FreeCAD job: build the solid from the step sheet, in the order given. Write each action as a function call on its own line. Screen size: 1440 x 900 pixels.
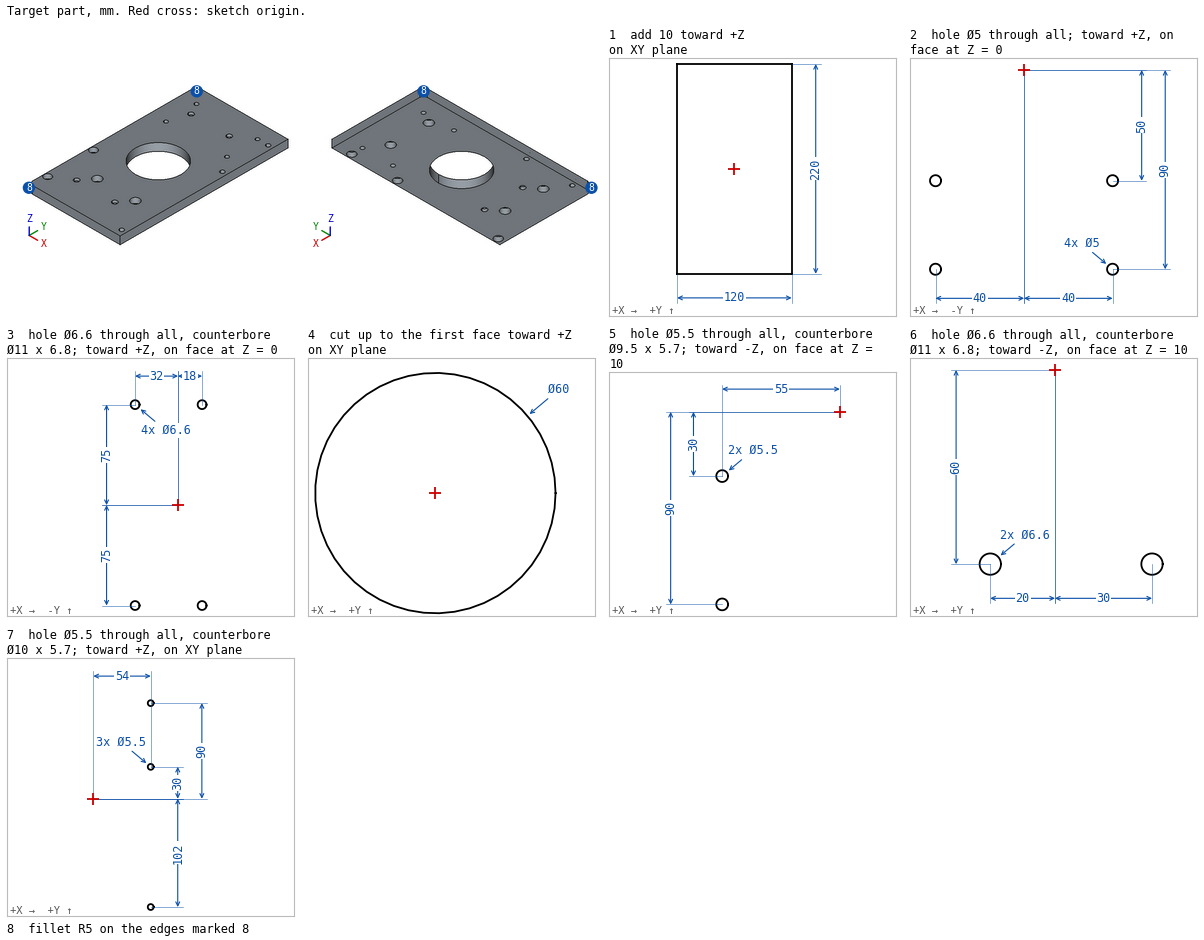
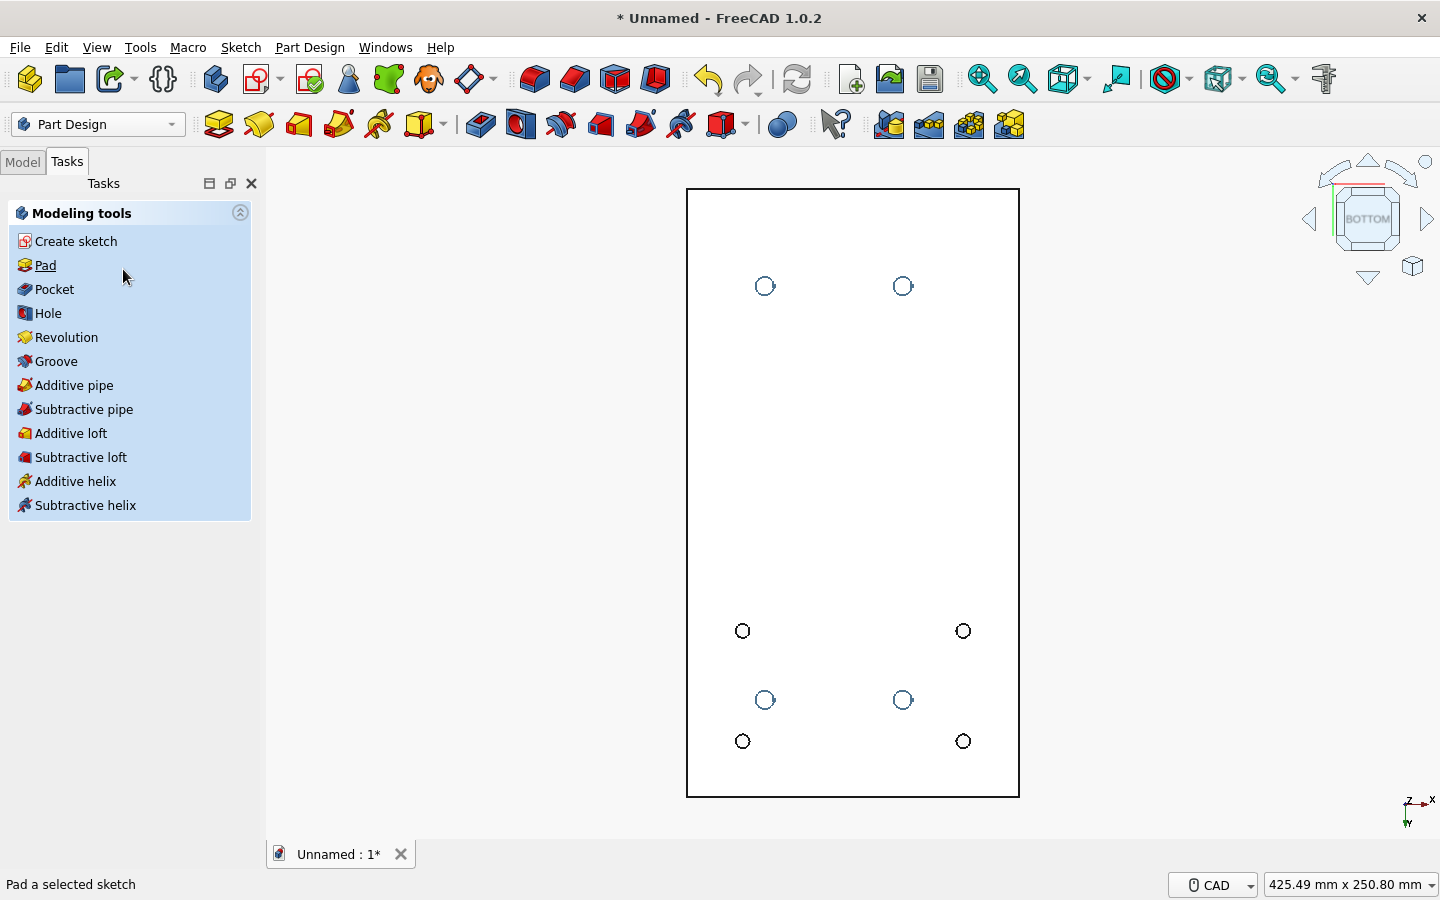
click(522, 124)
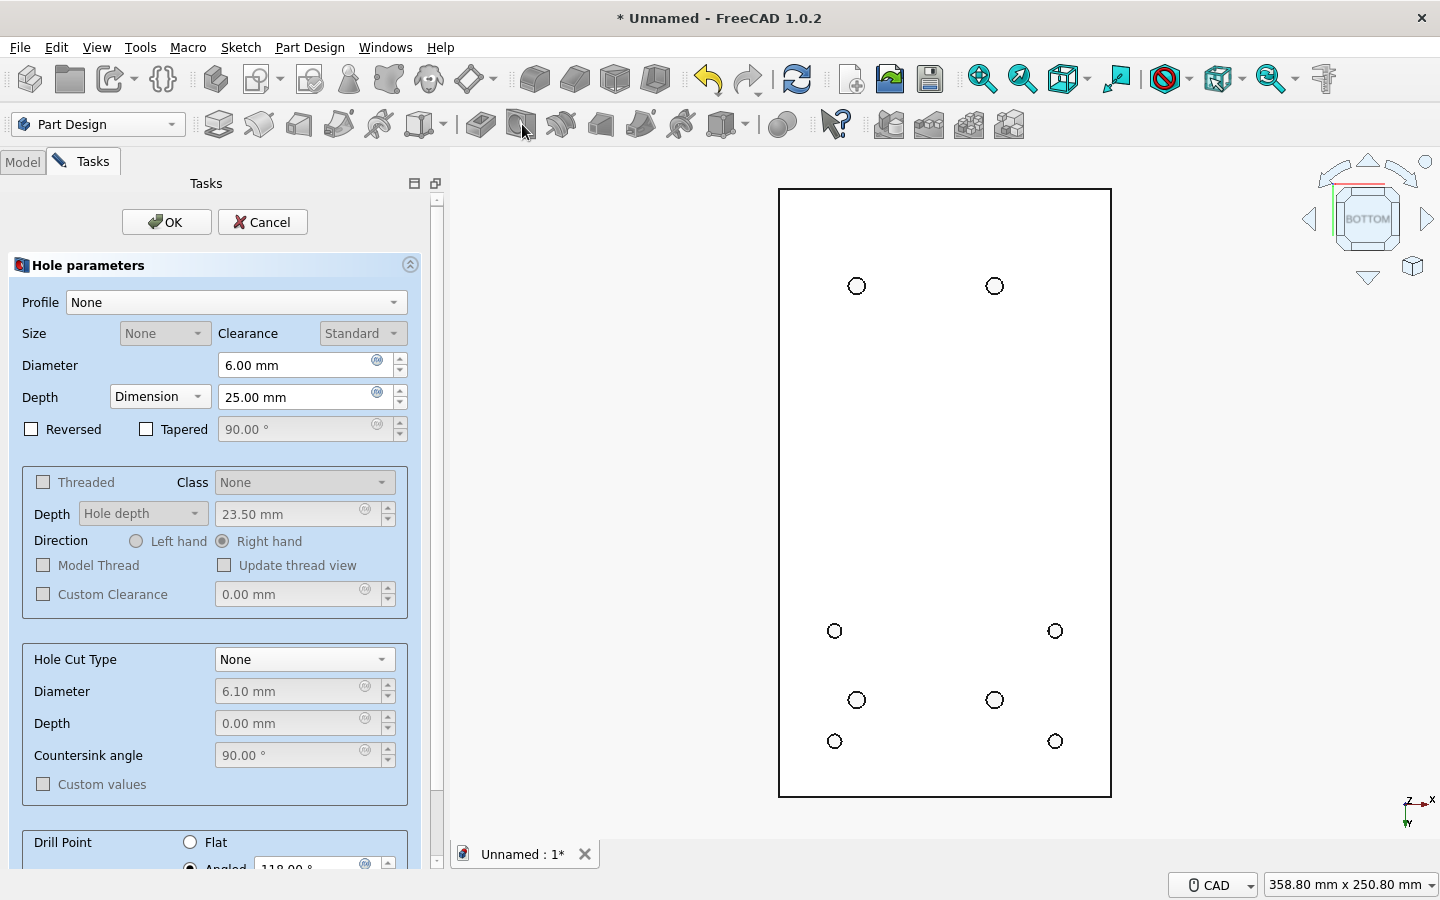
triple_click(305, 365)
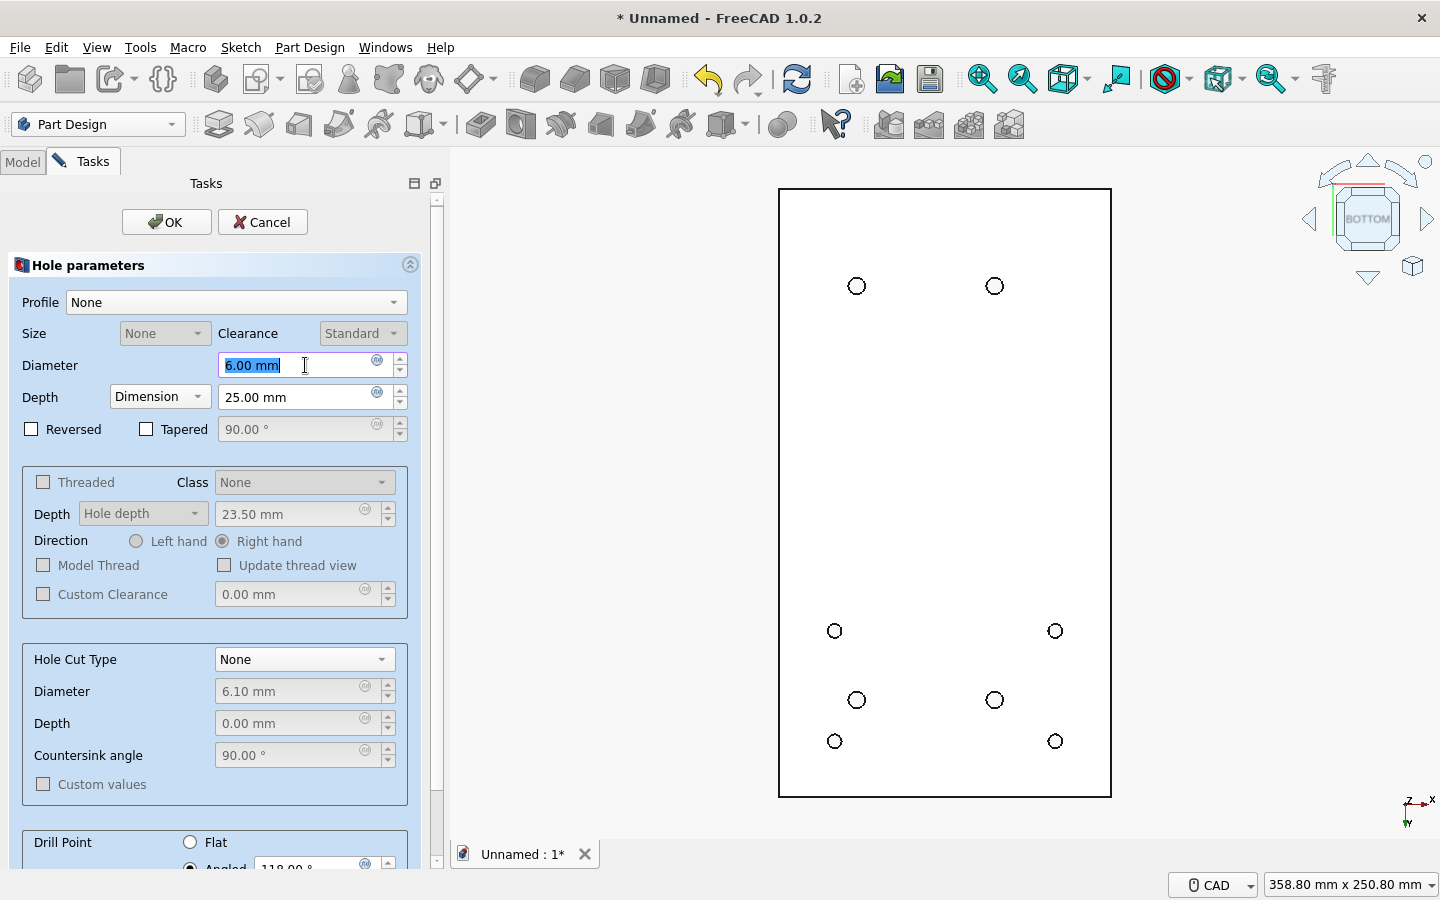
text(6.6)
key(Tab)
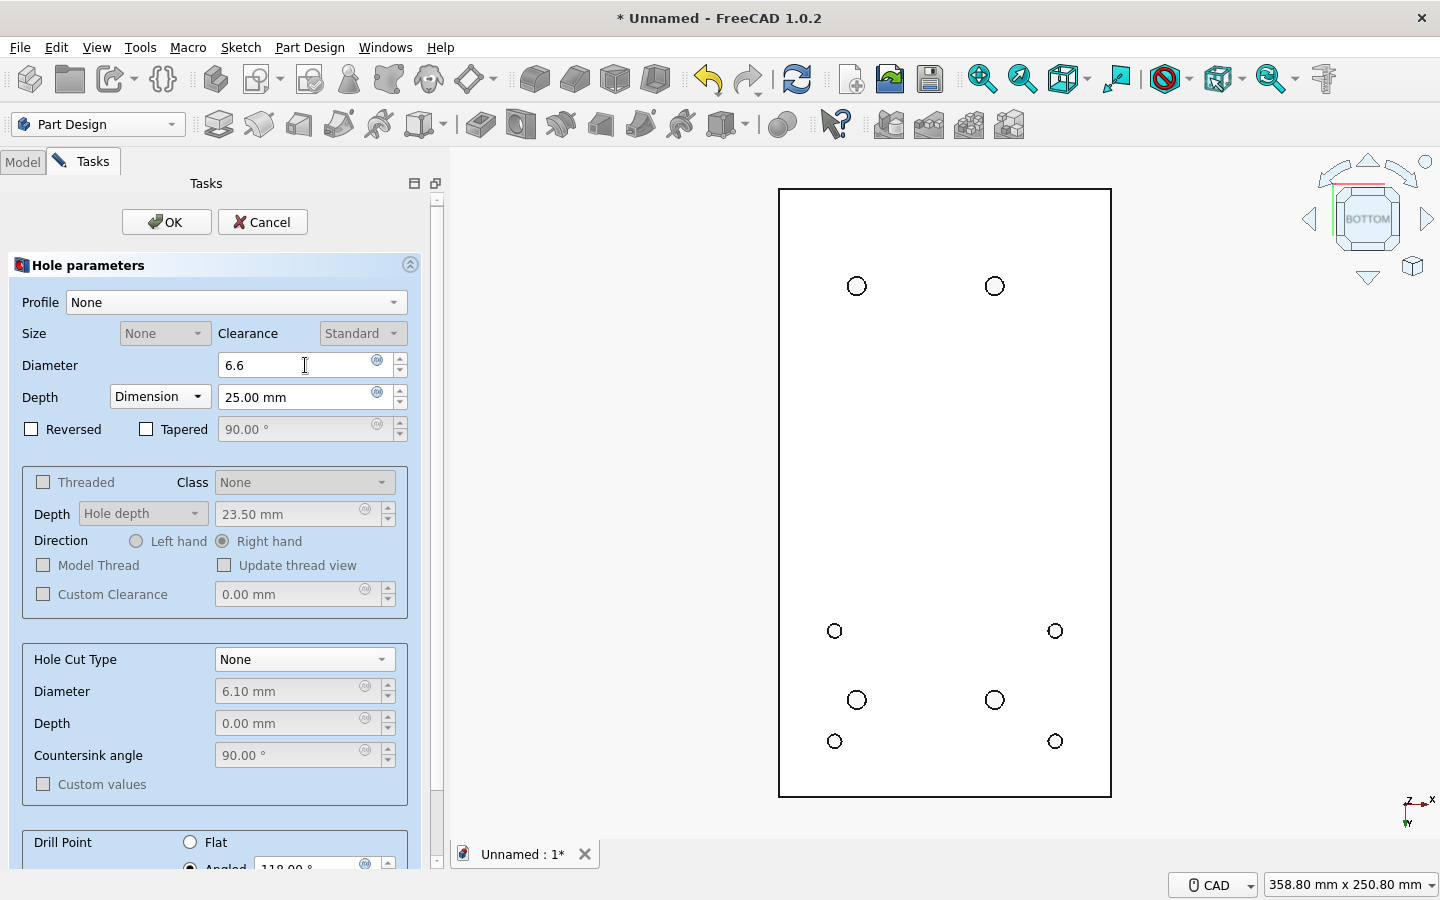
click(161, 396)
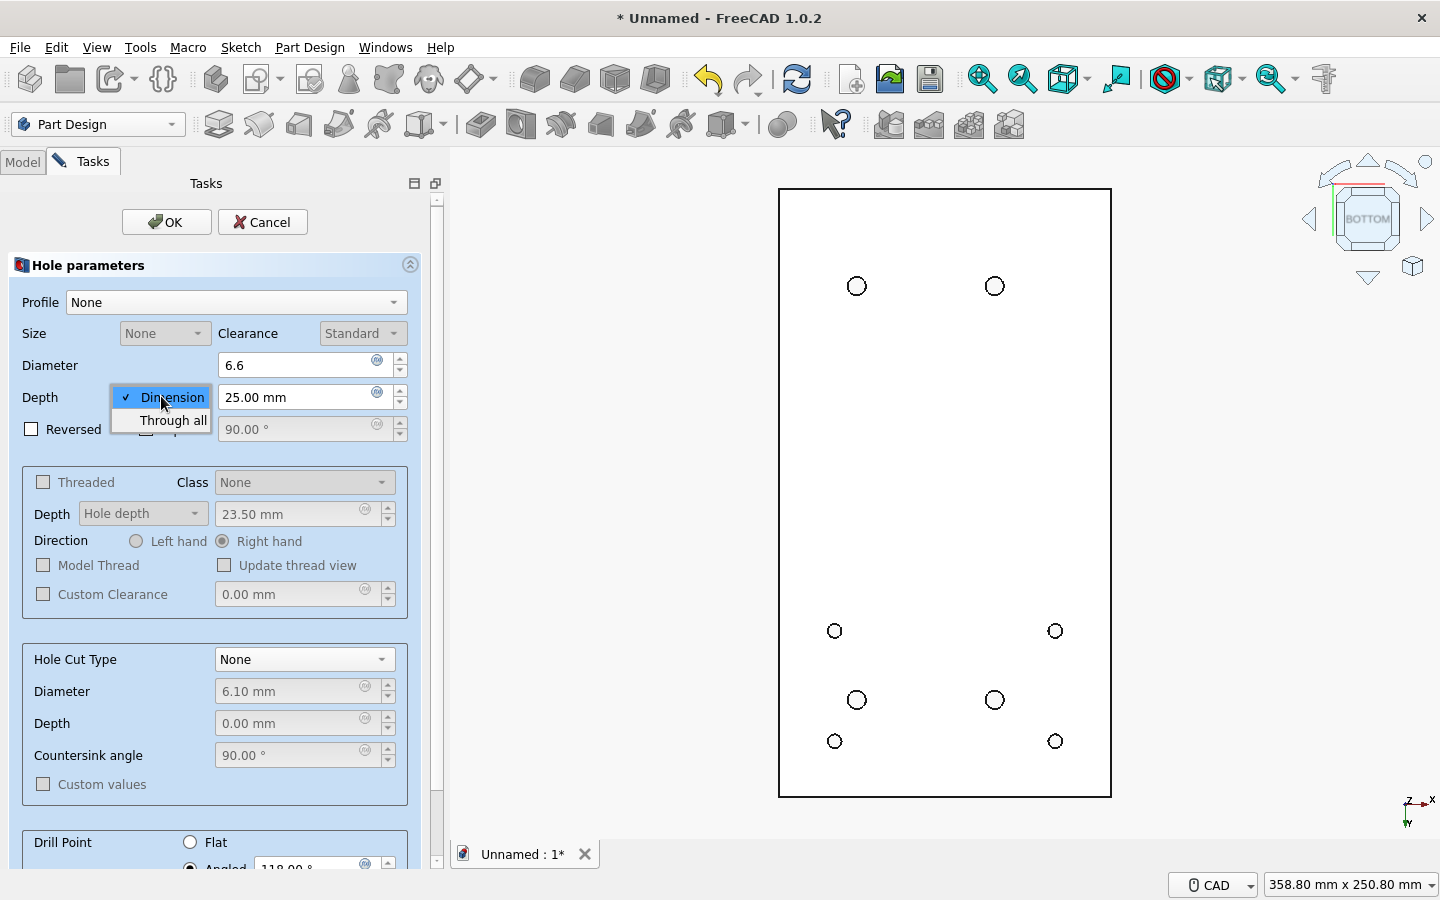
click(160, 420)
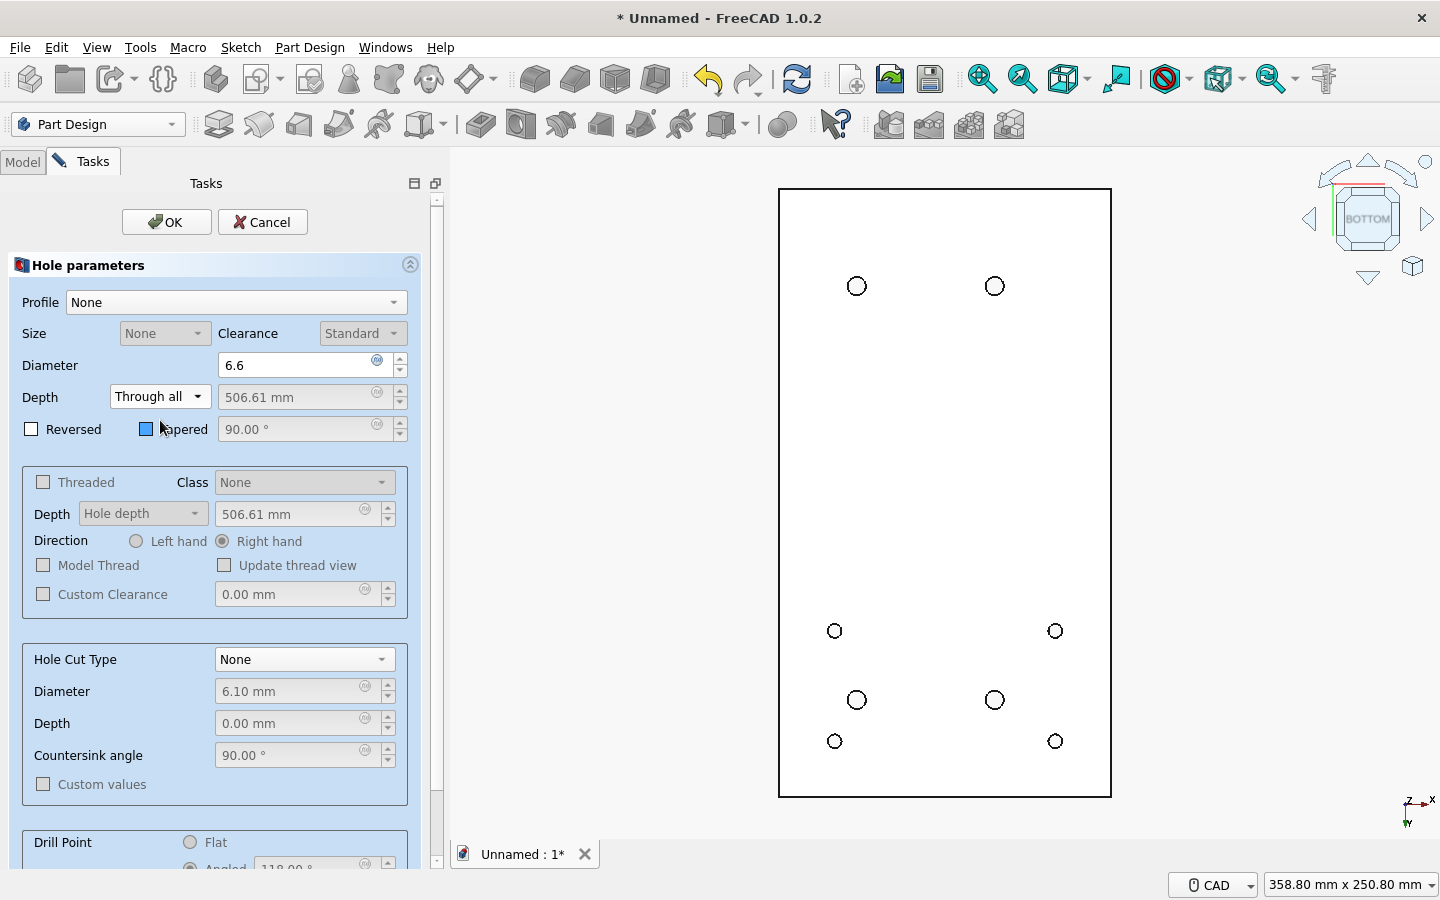
click(306, 660)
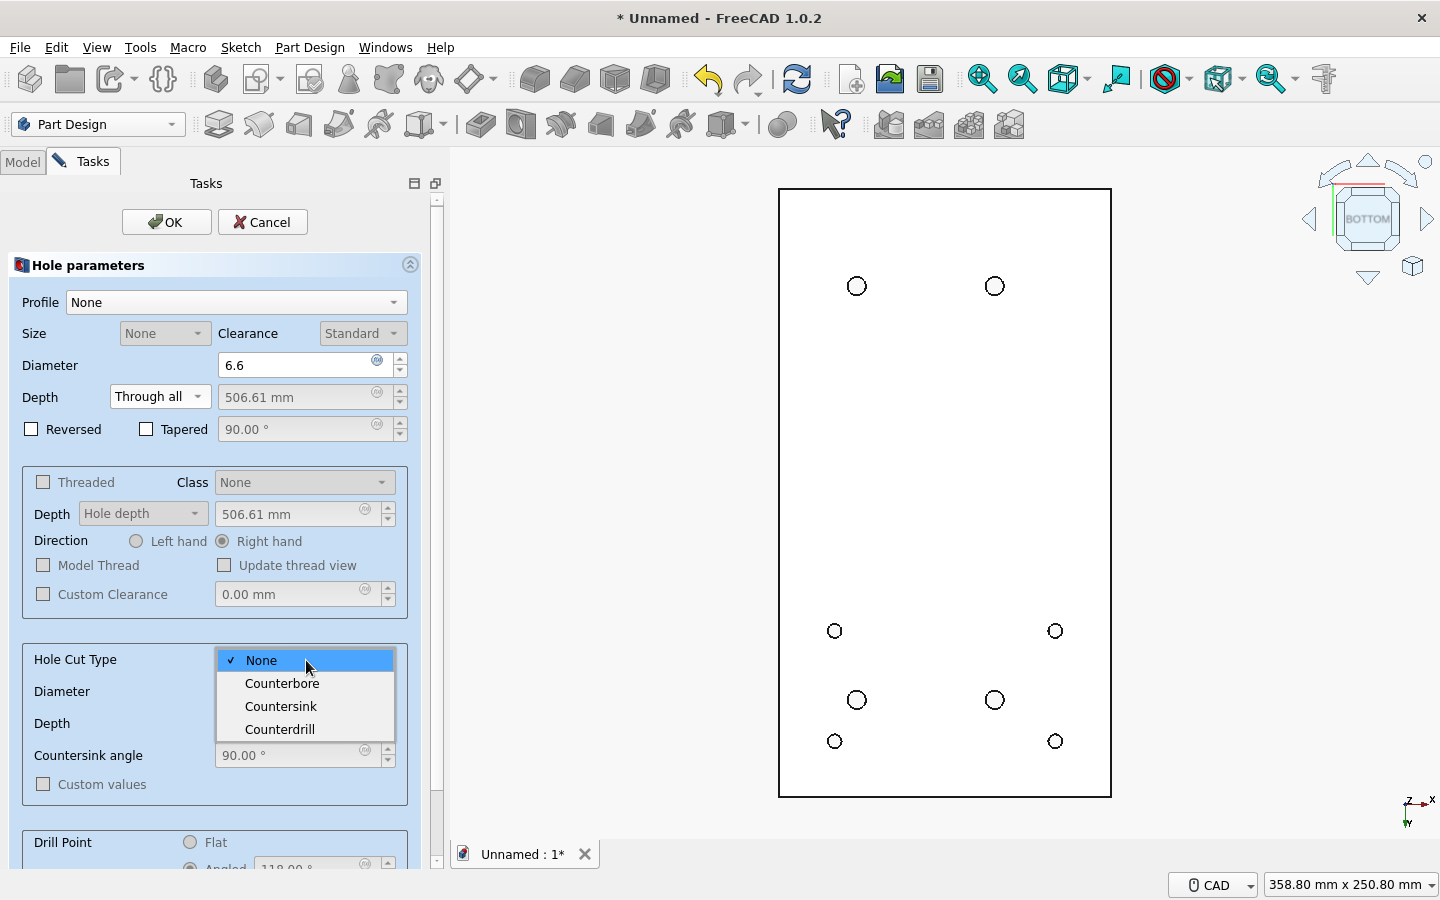
click(304, 684)